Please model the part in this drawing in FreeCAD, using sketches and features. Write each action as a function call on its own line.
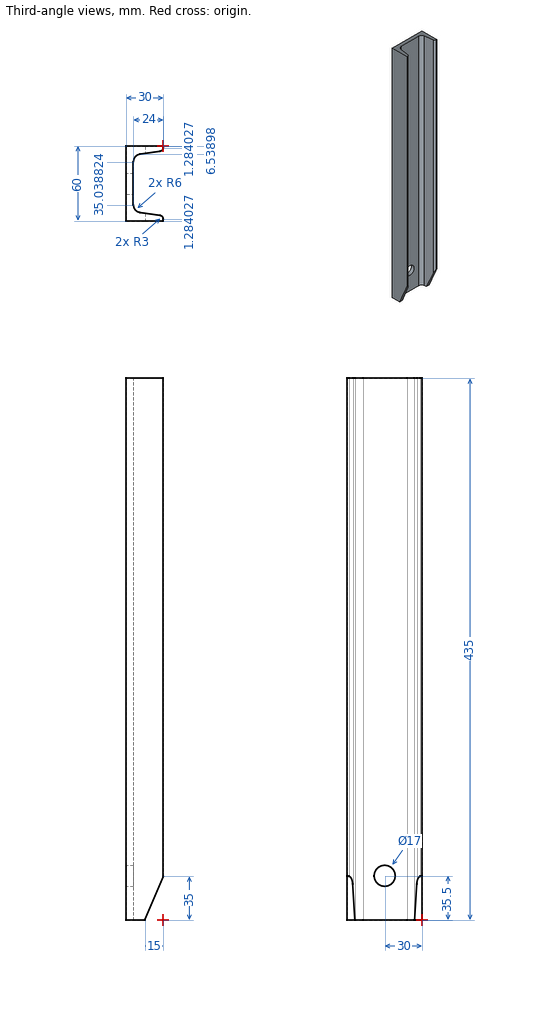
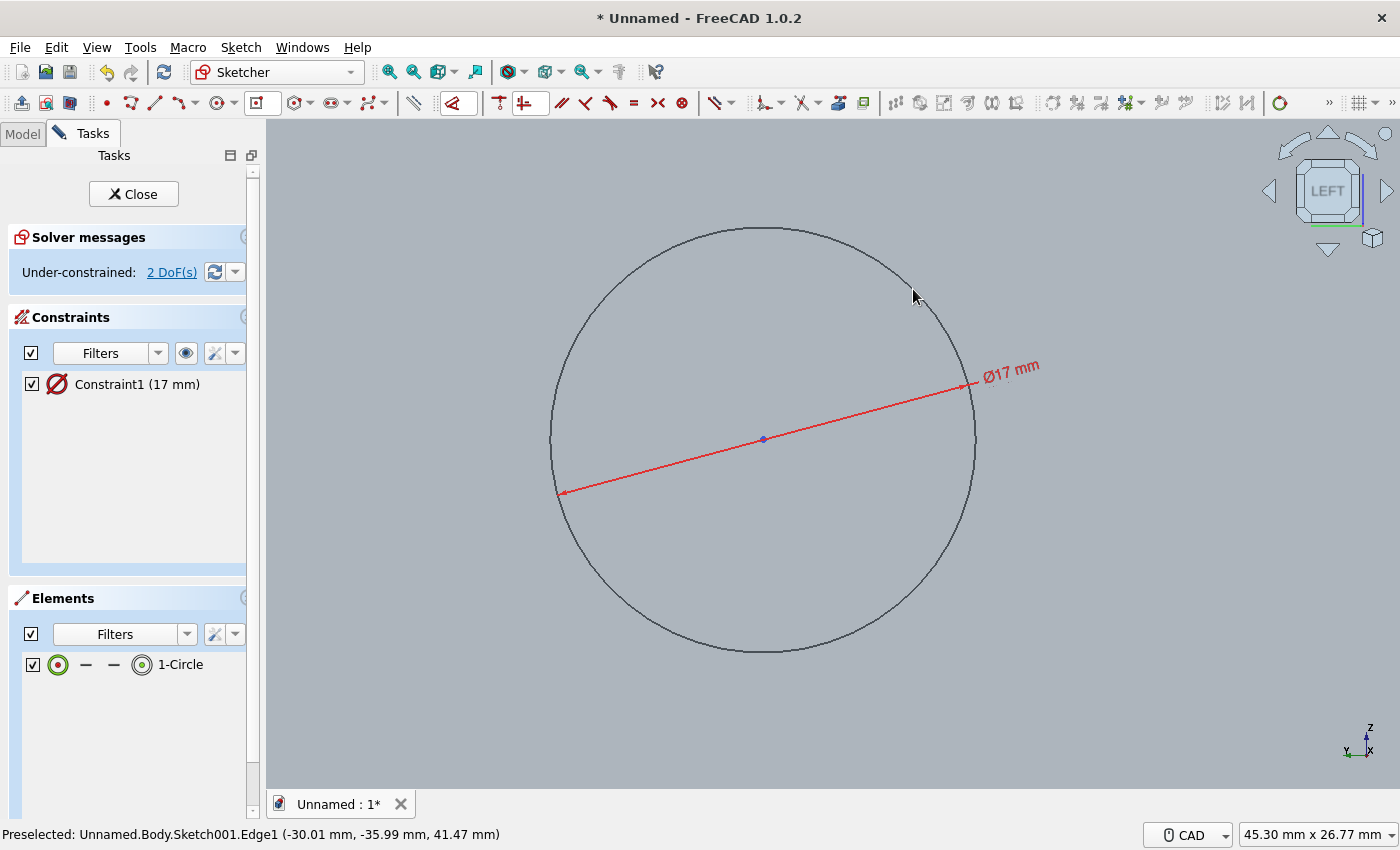
click(763, 440)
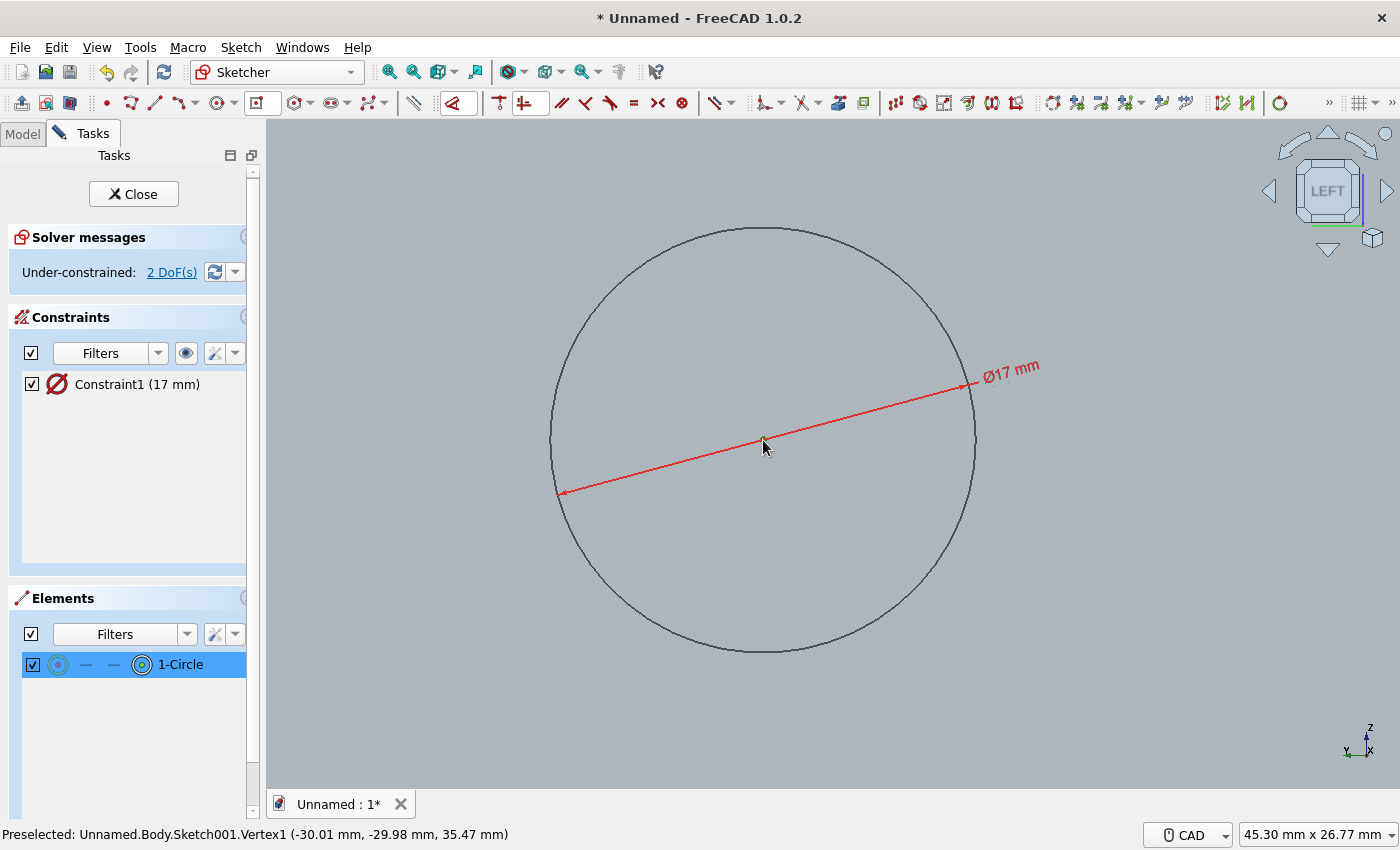
click(472, 104)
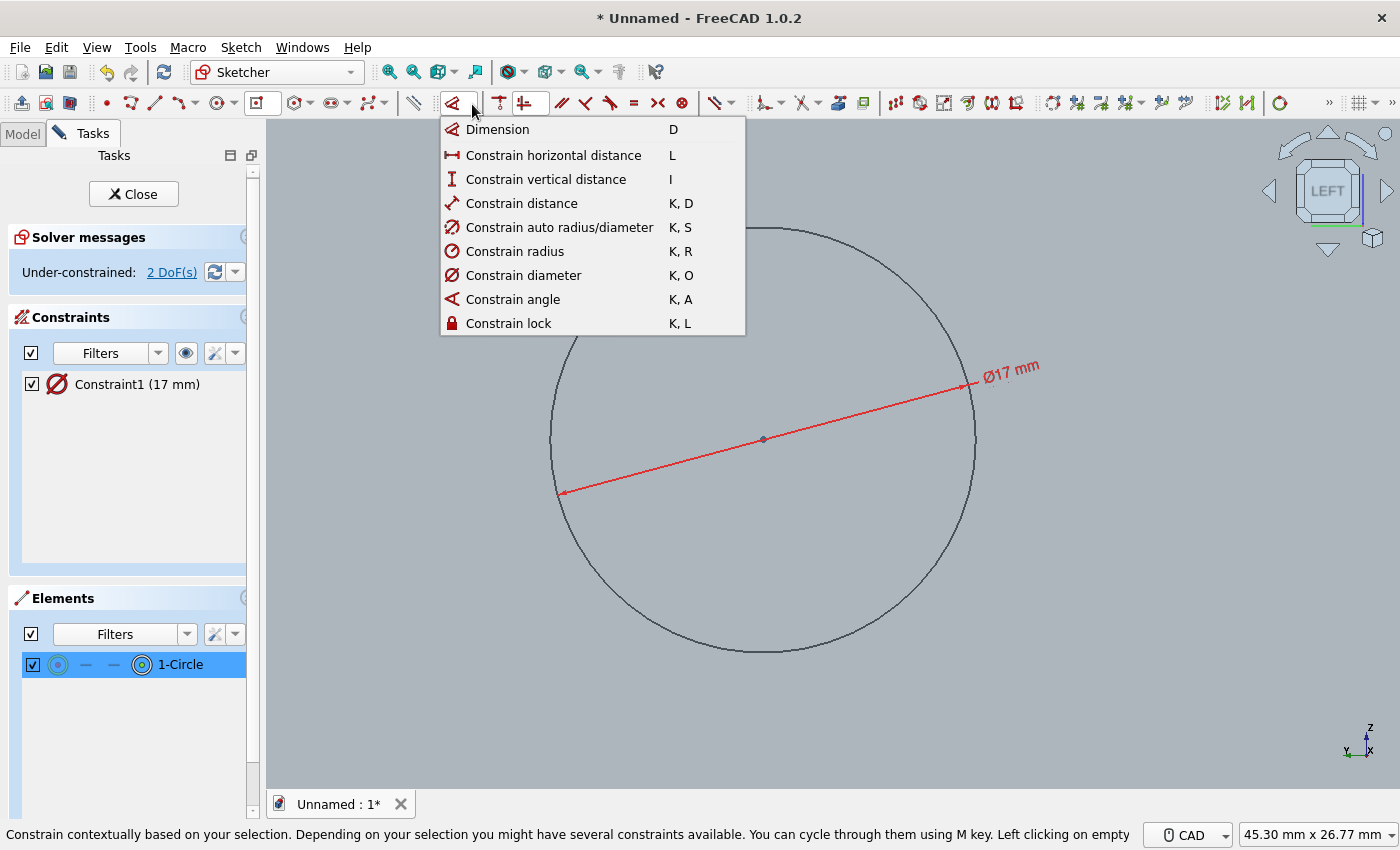
click(593, 155)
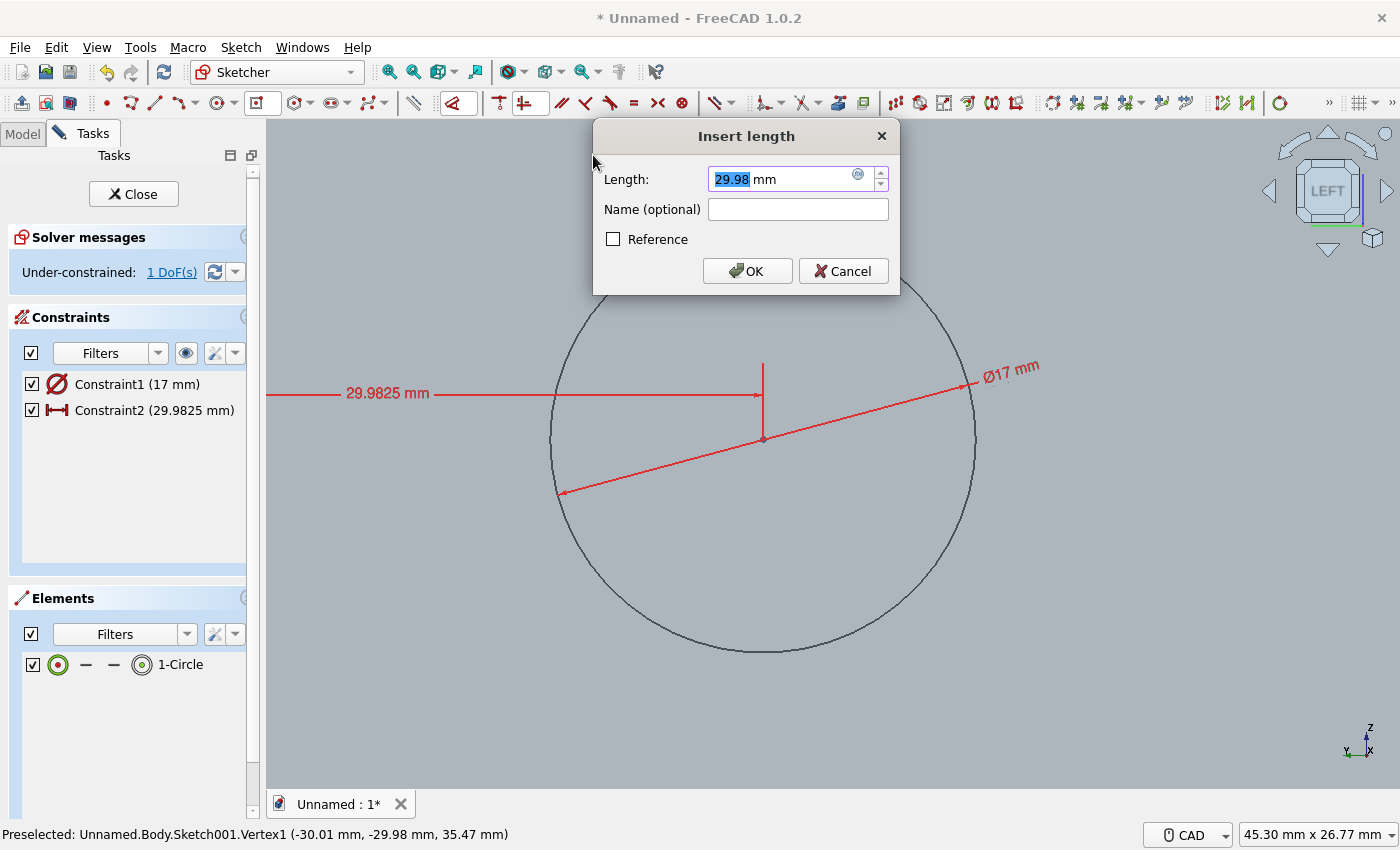
text(30)
key(Return)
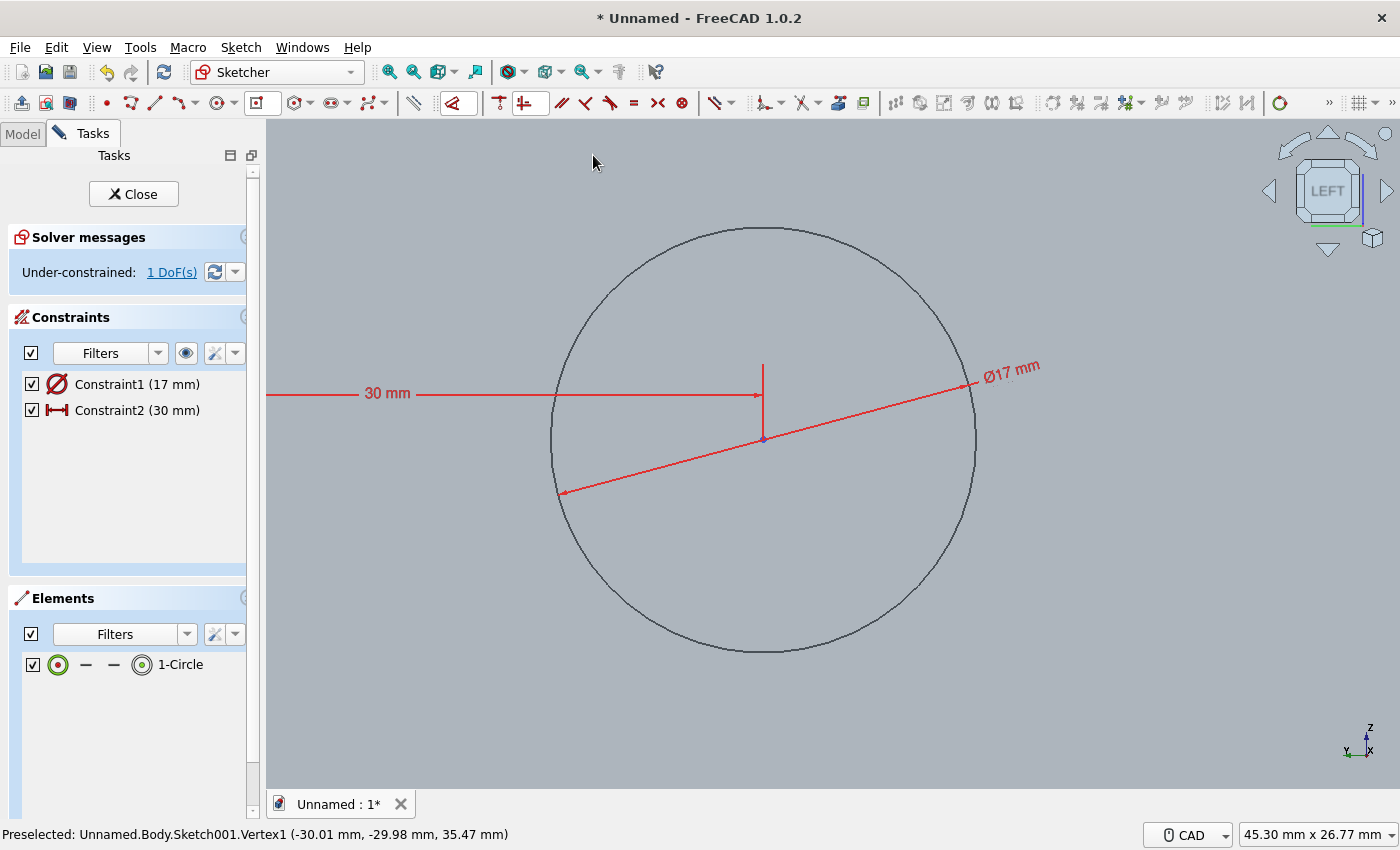
click(763, 440)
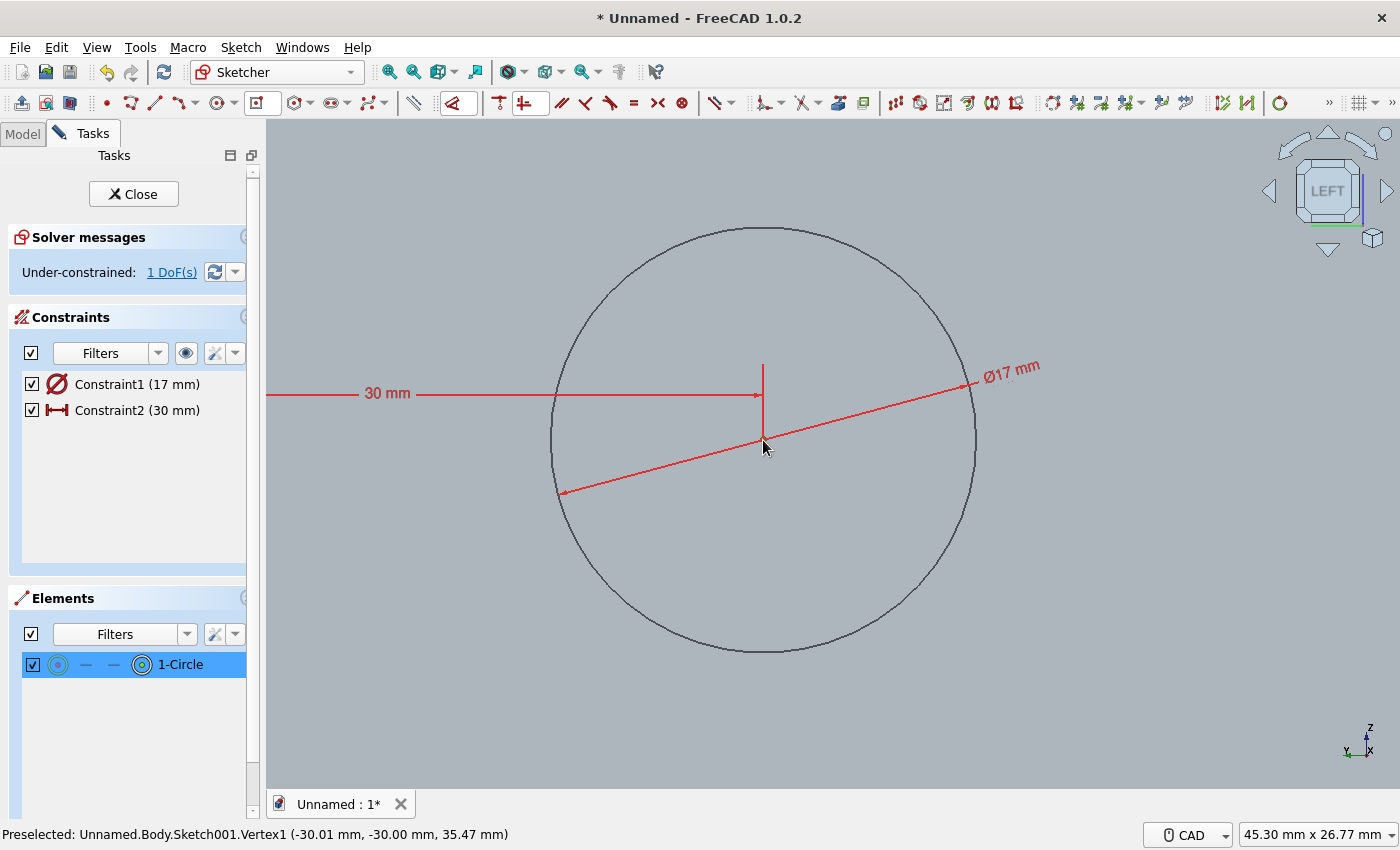
click(472, 104)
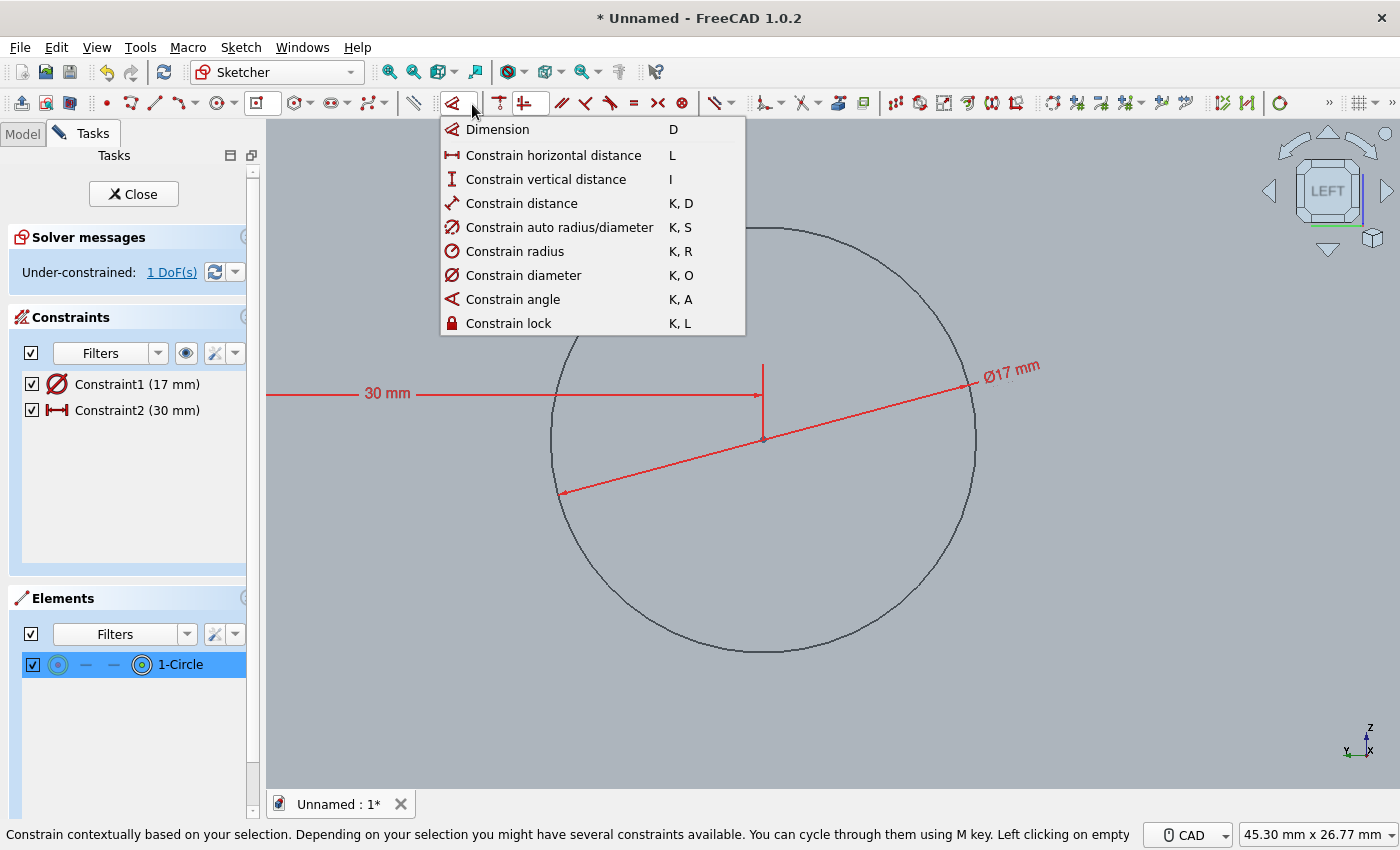
click(593, 179)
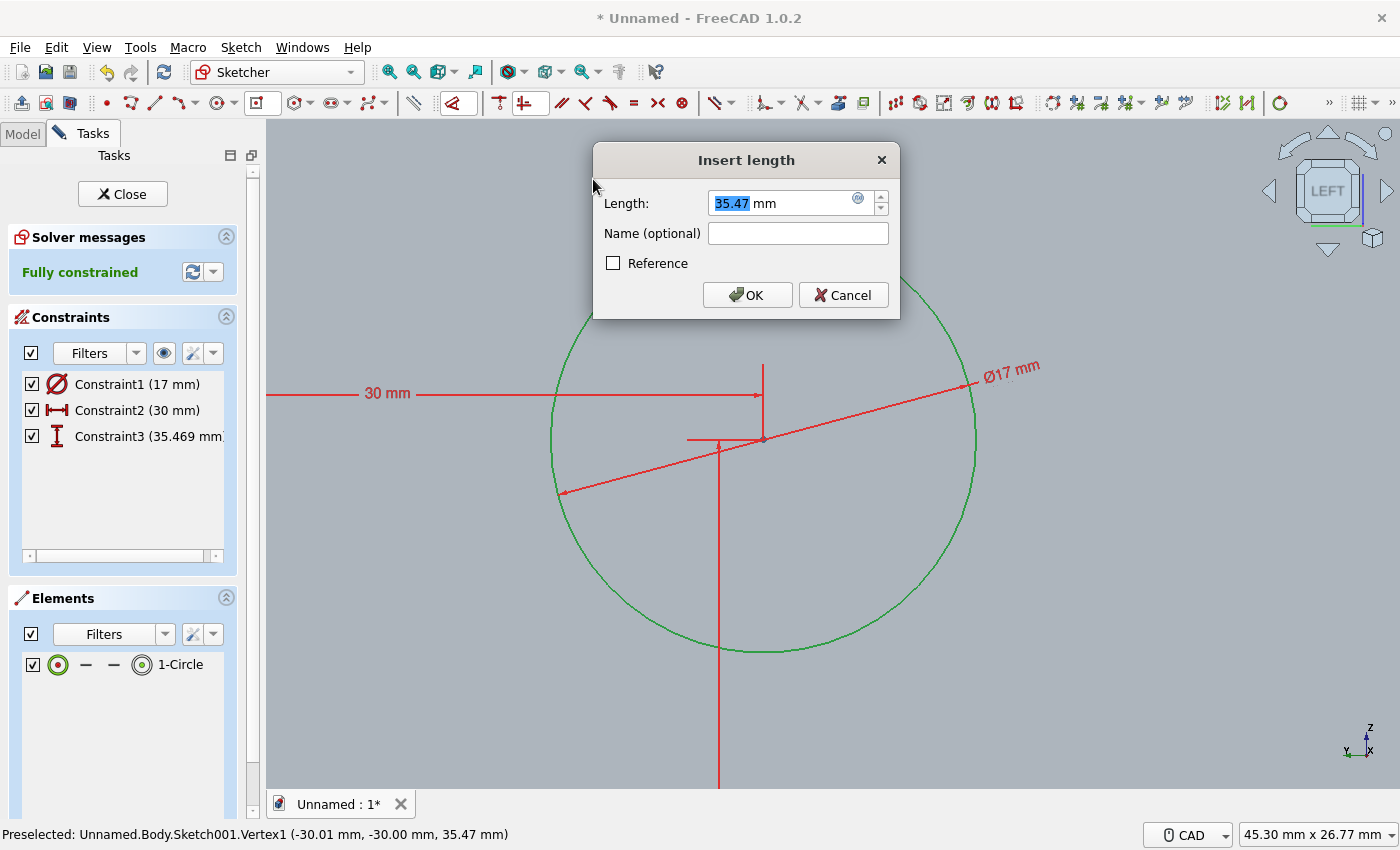
text(35.5)
key(Return)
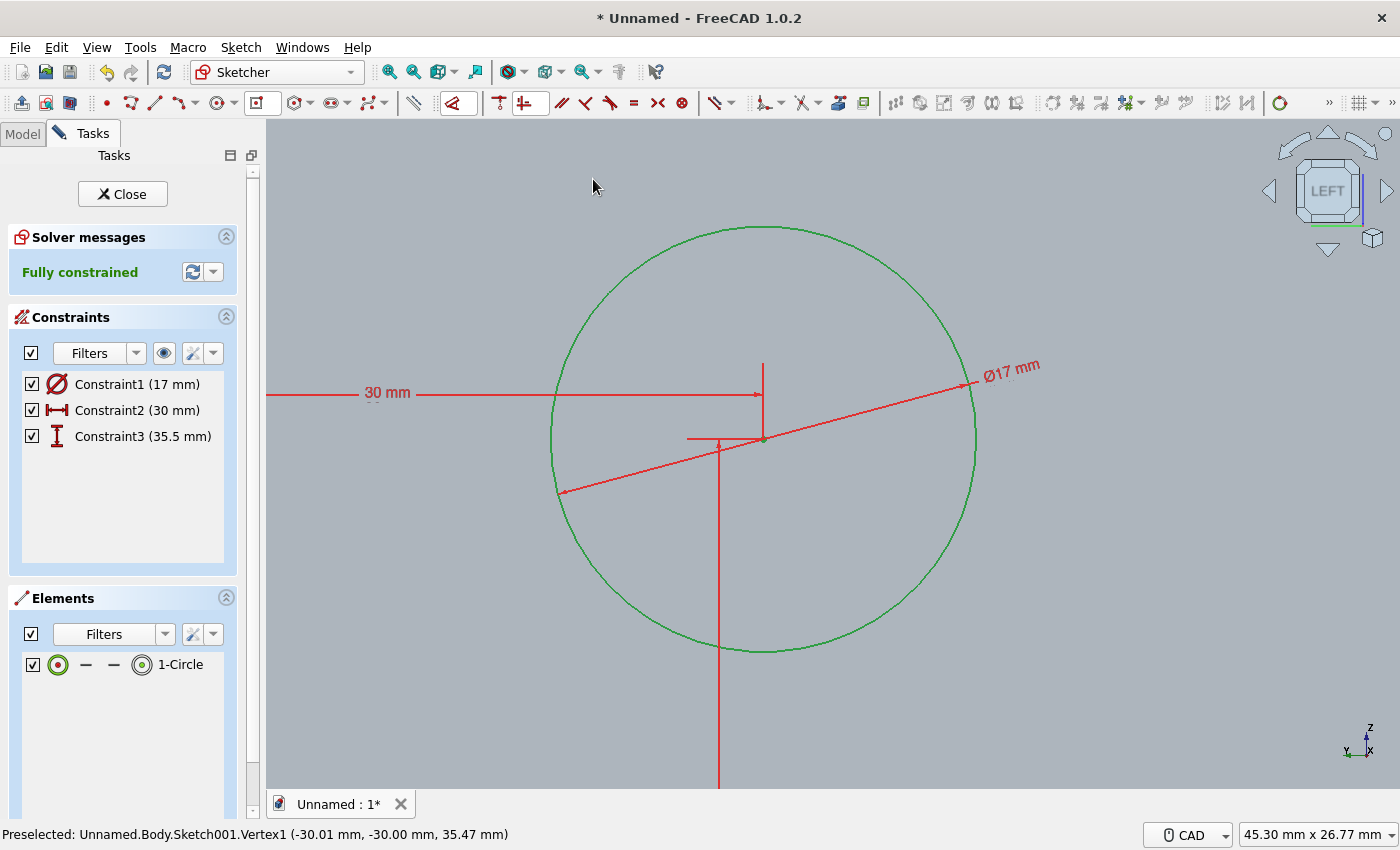
click(123, 194)